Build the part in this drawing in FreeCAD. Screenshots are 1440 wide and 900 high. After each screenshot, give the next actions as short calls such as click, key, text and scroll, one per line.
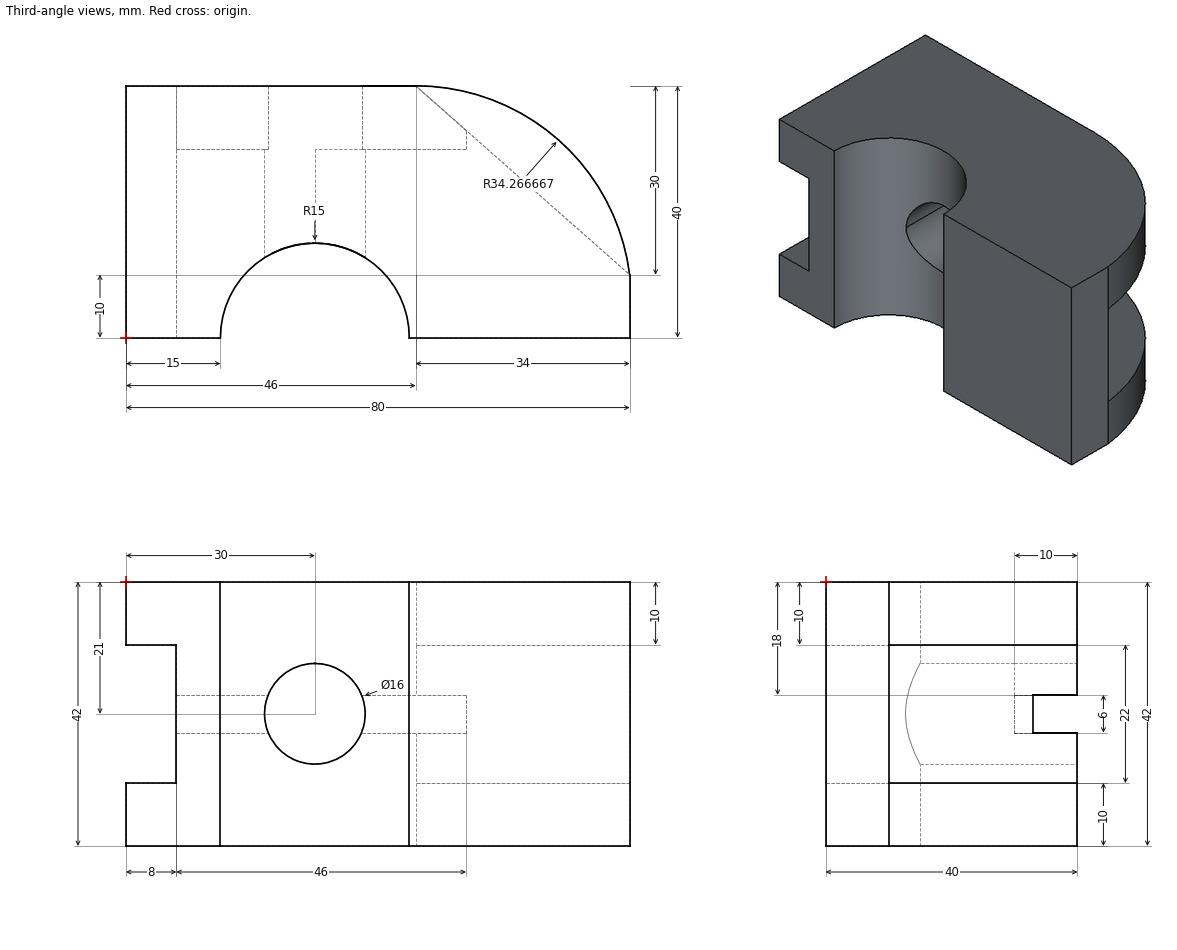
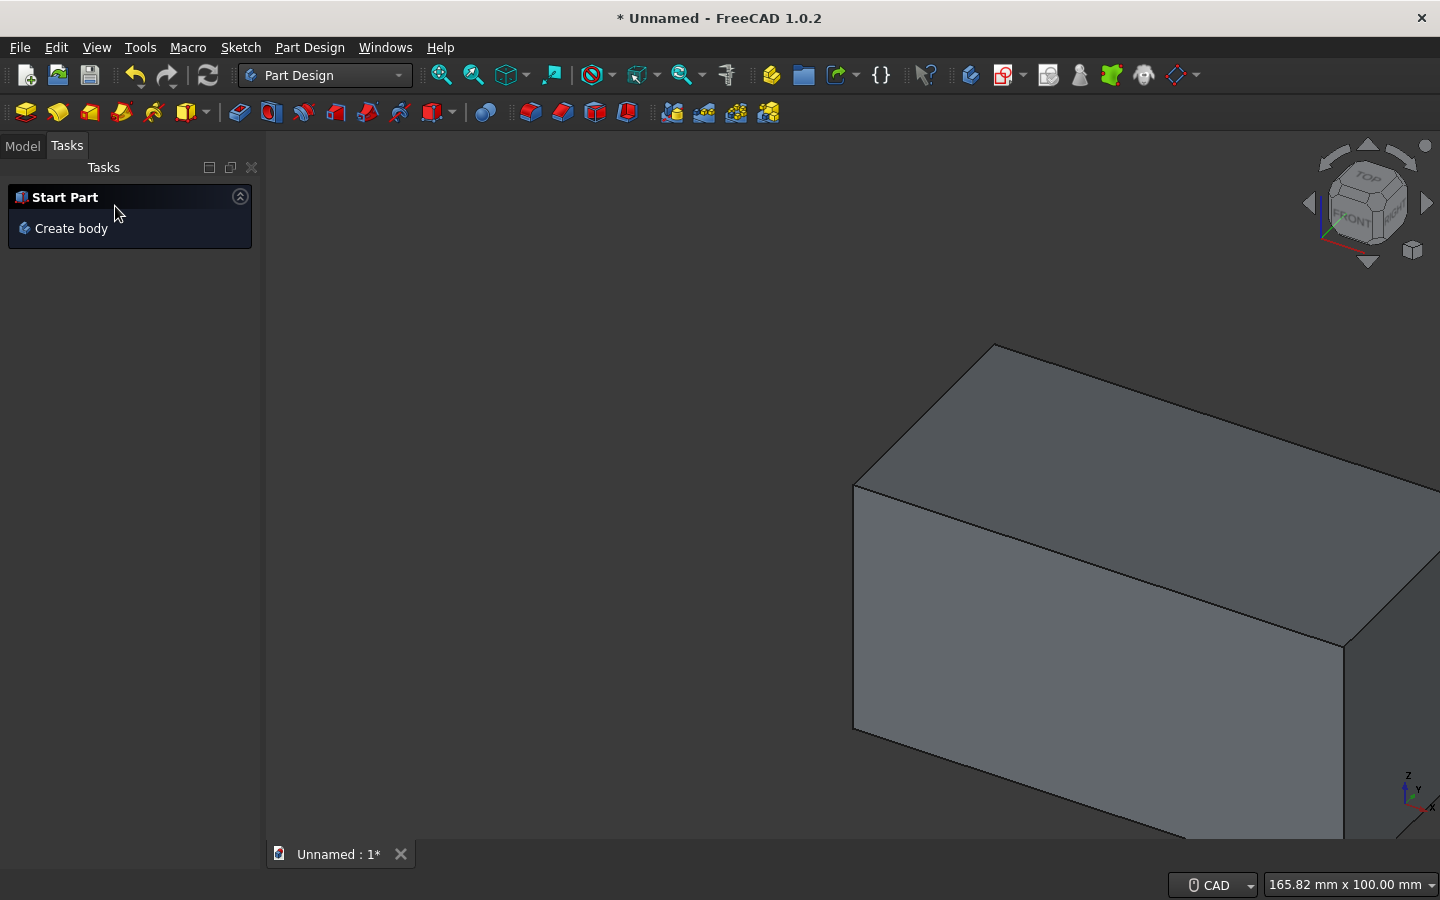
click(442, 76)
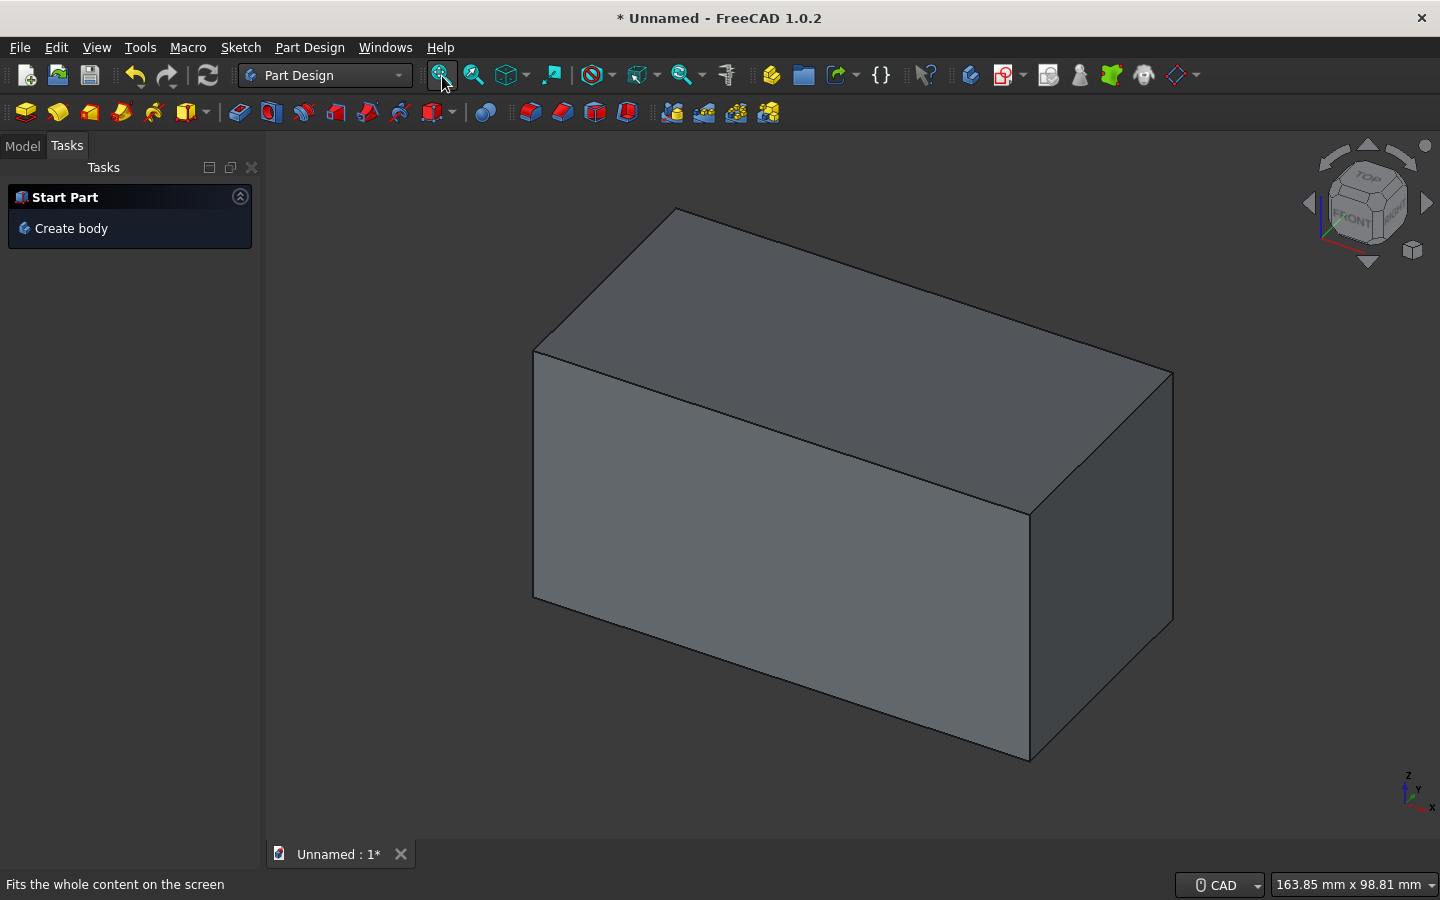
click(924, 384)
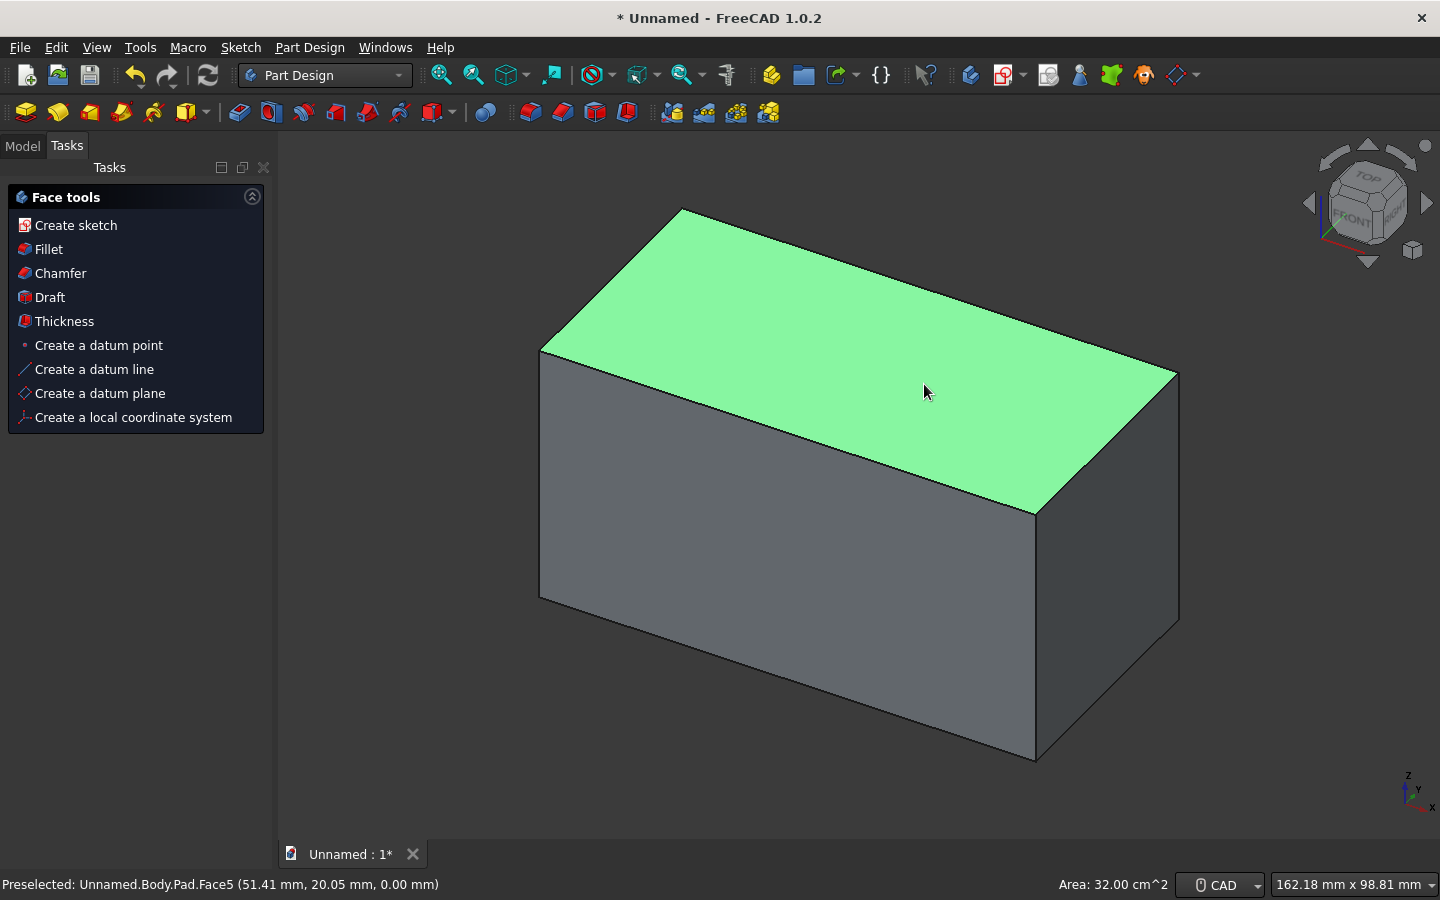
click(1004, 76)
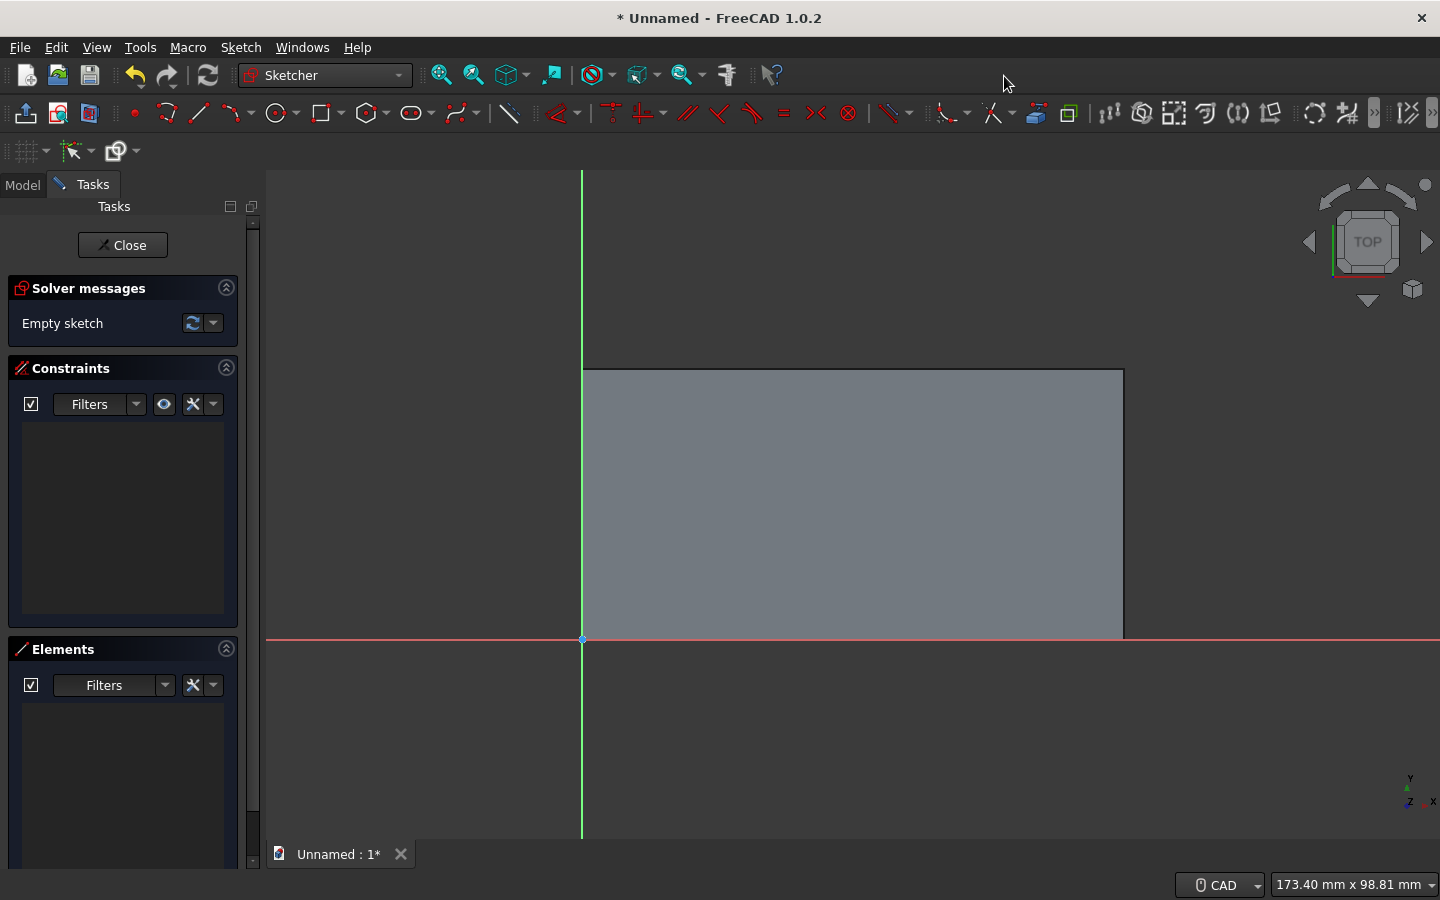
click(322, 114)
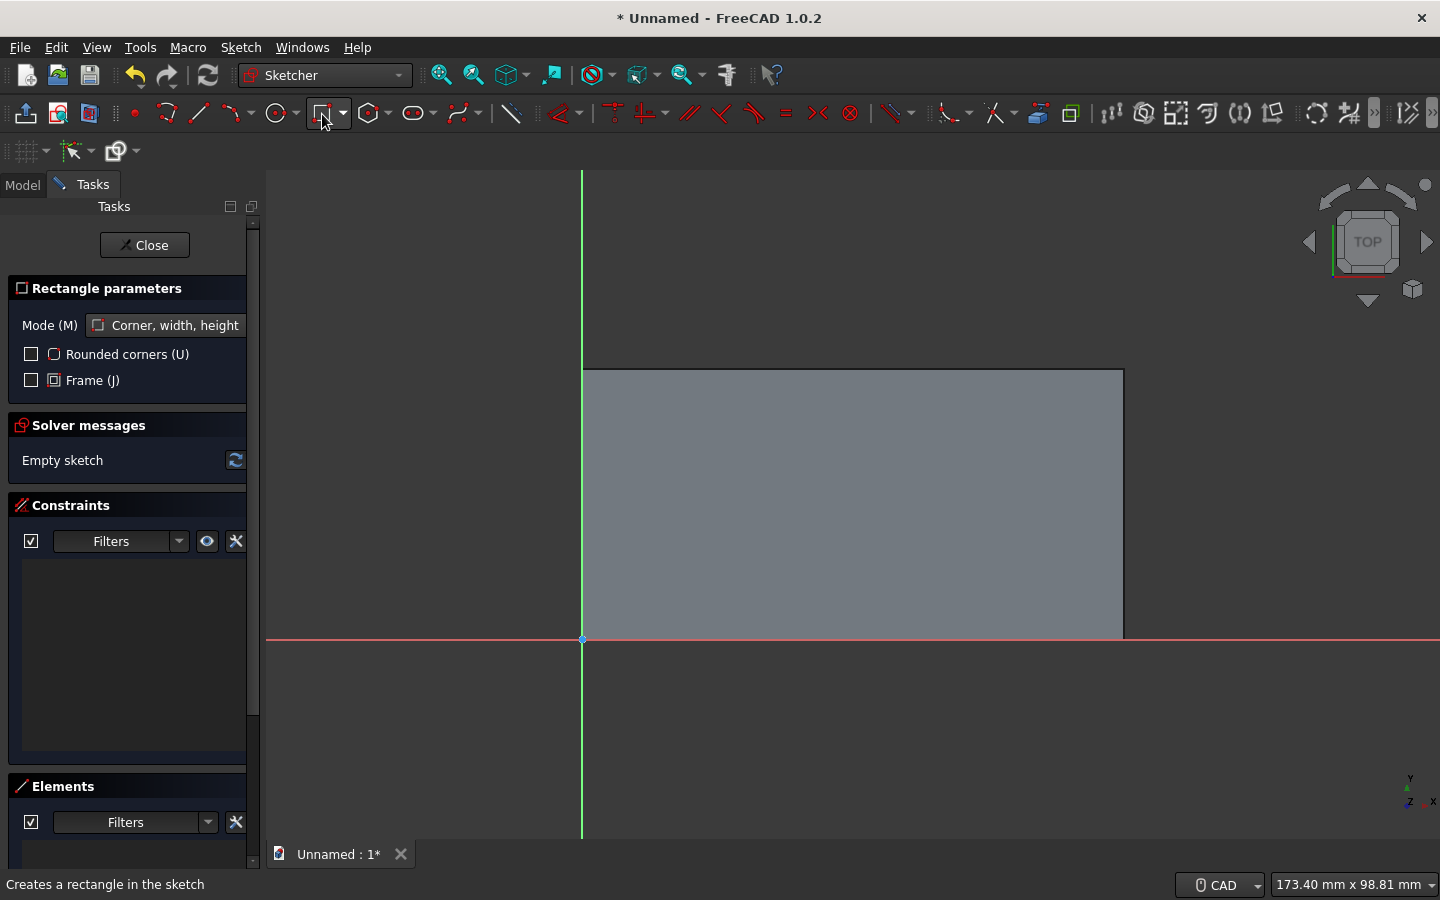
click(894, 369)
move(1124, 572)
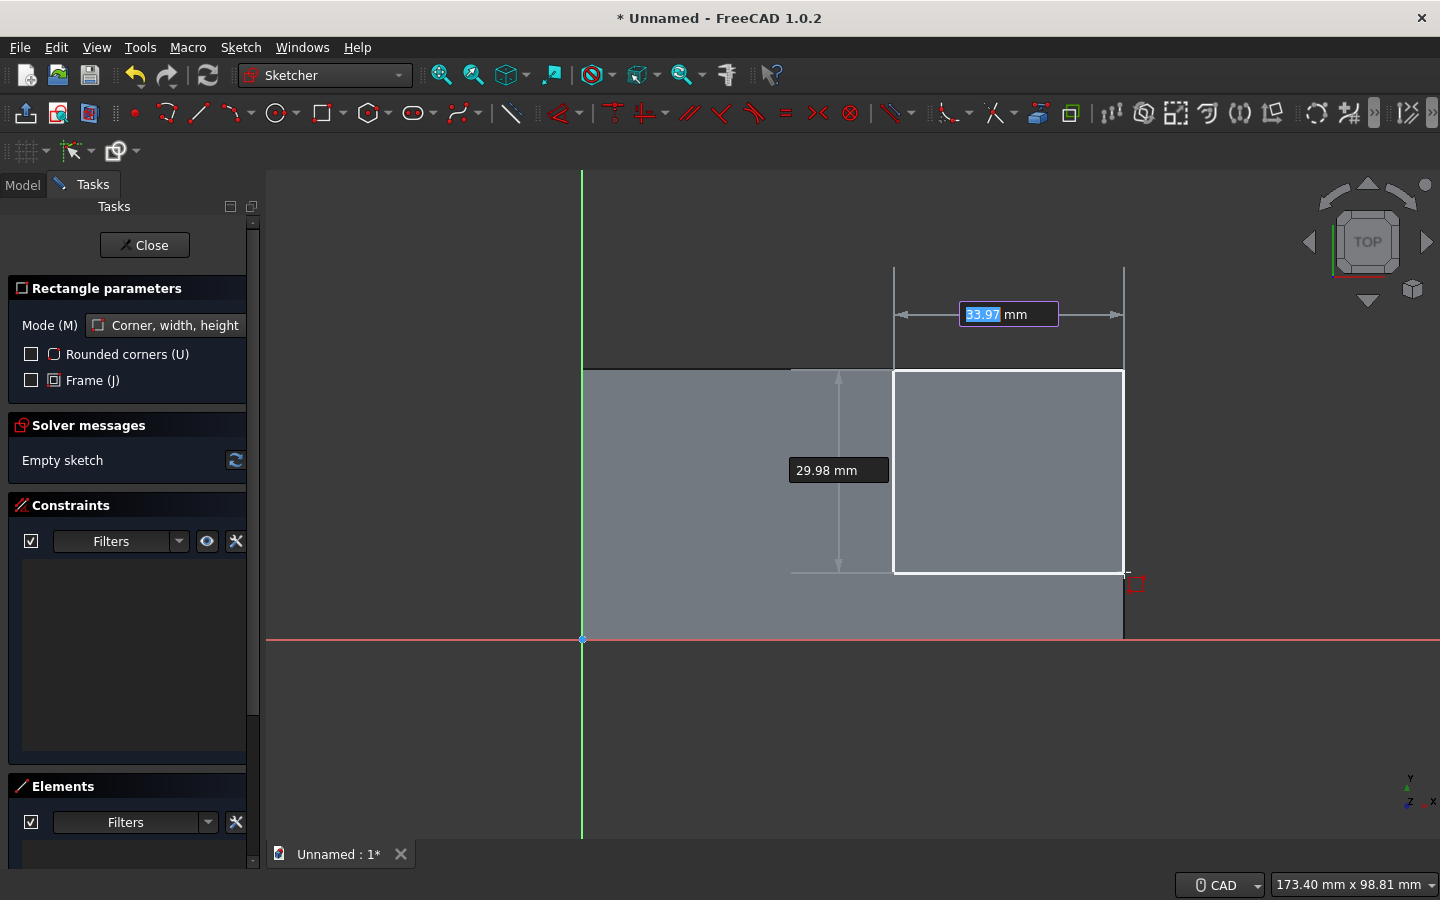
text(34)
key(Tab)
text(30)
key(Return)
key(Escape)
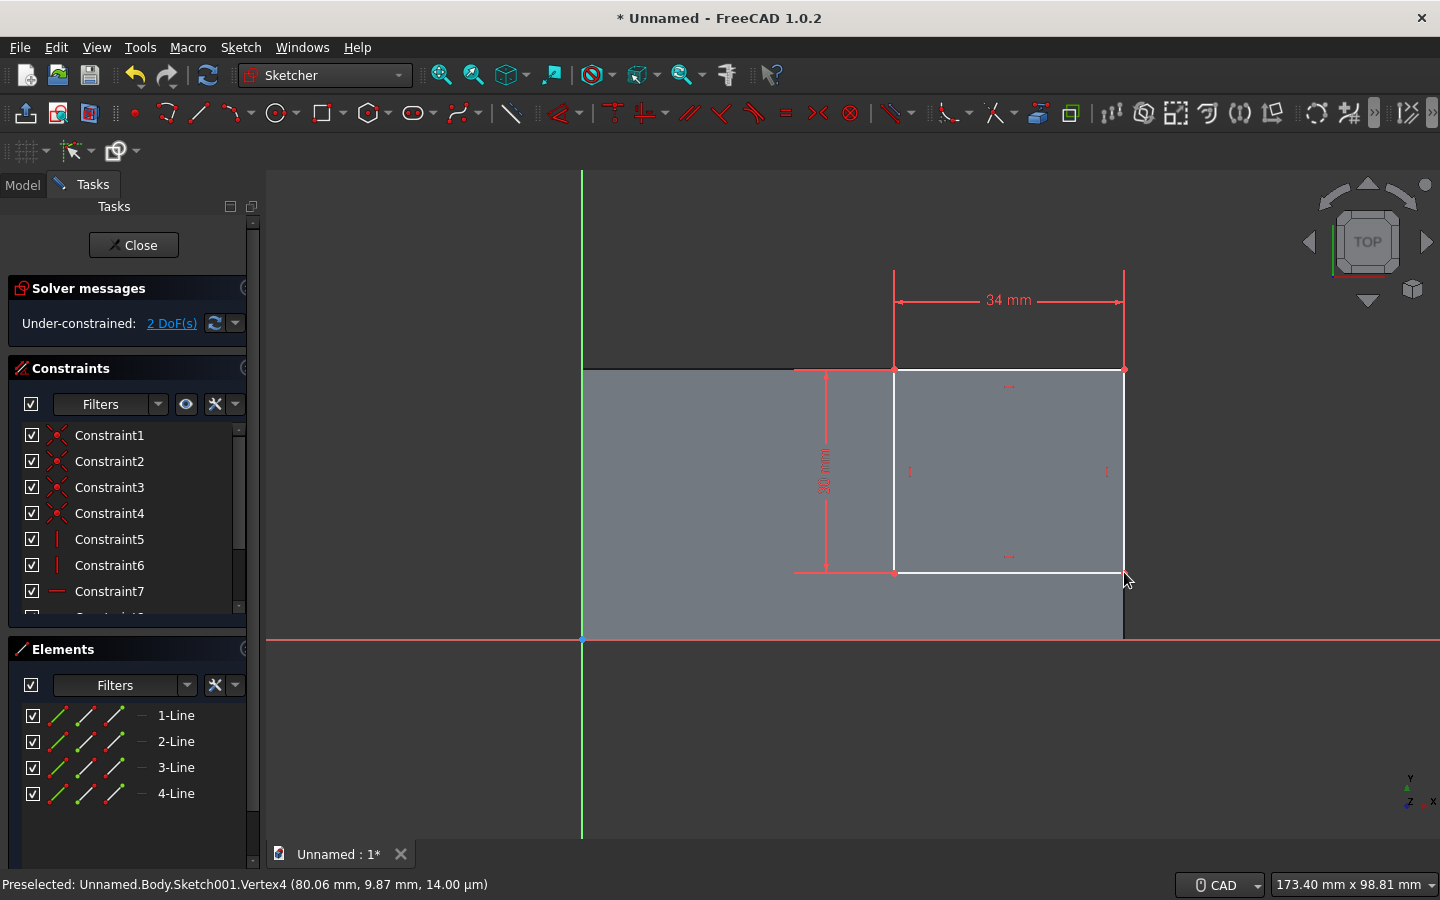
click(894, 370)